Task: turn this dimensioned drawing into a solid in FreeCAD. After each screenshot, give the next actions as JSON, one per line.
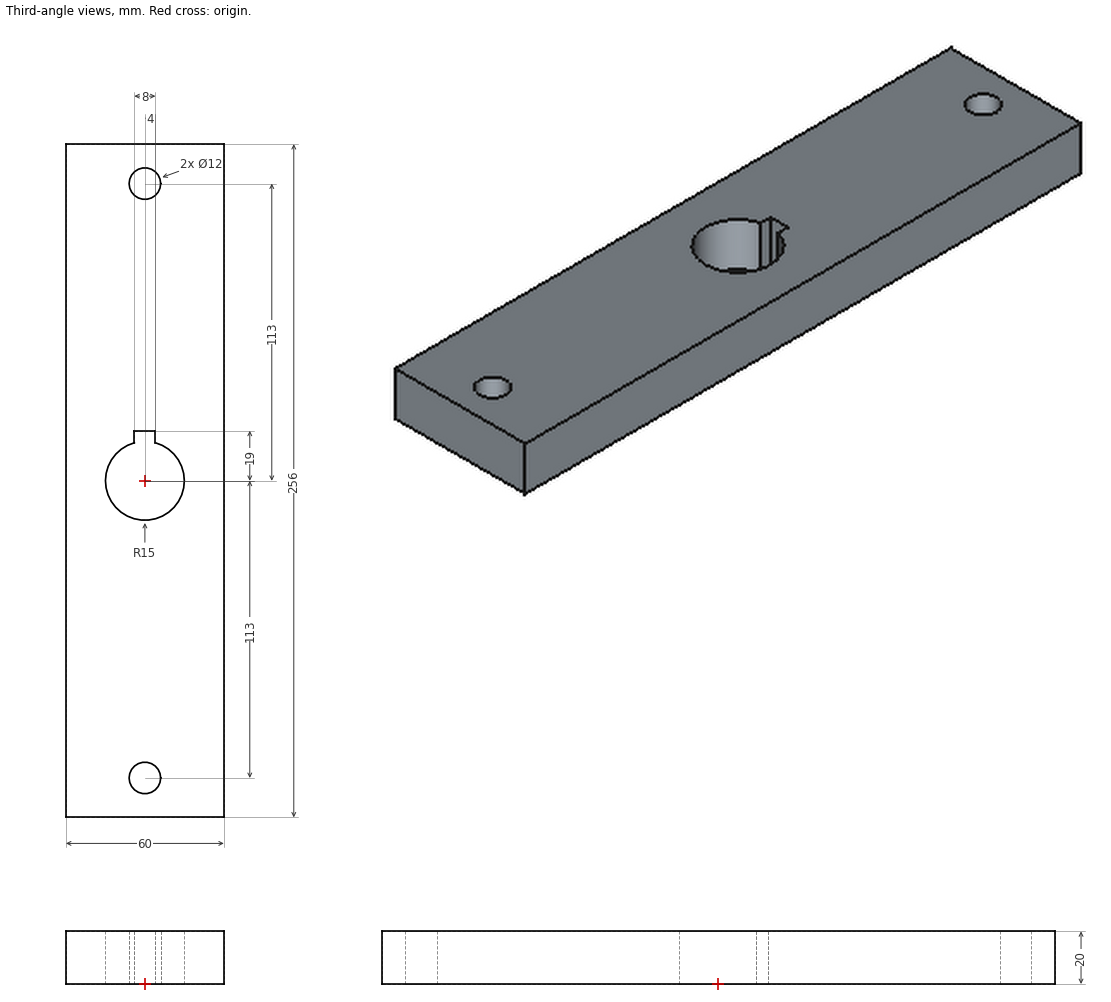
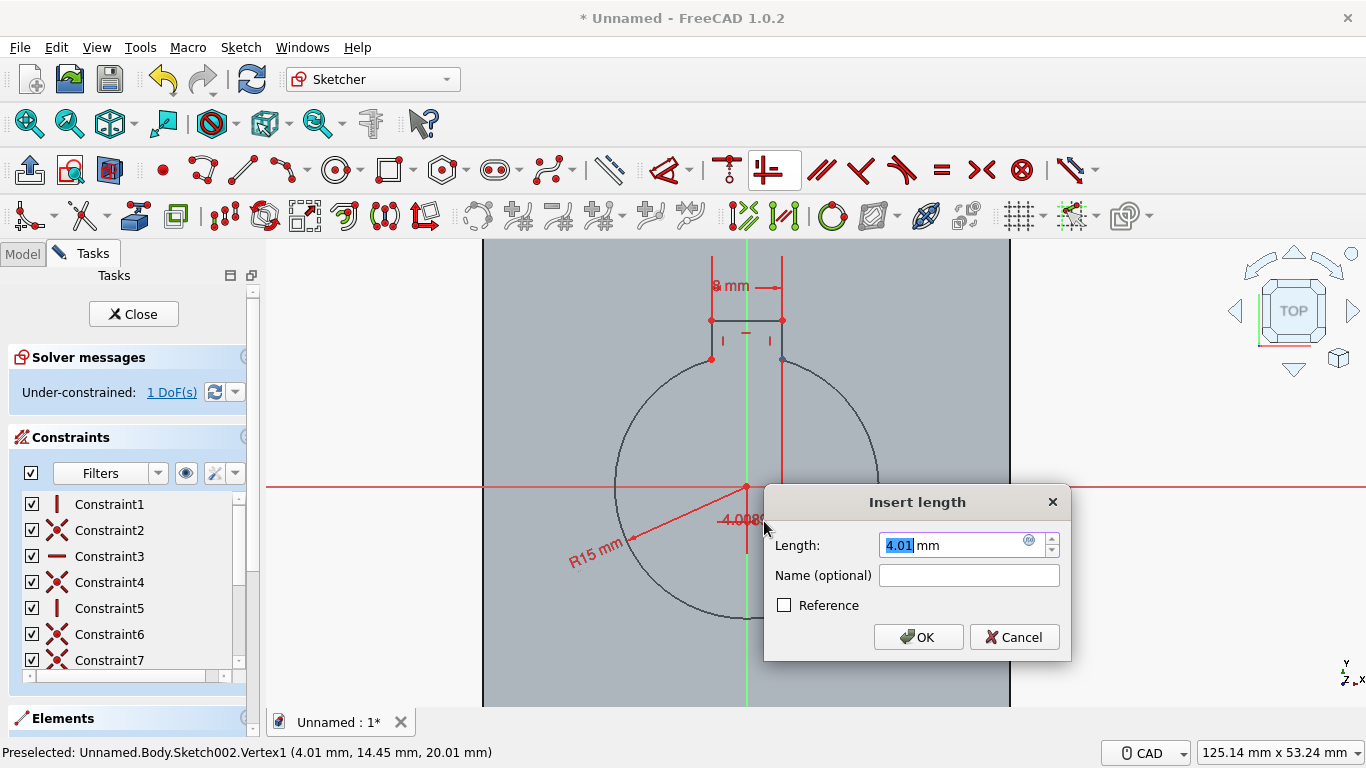
{"action": "type", "text": "4"}
{"action": "key", "text": "Return"}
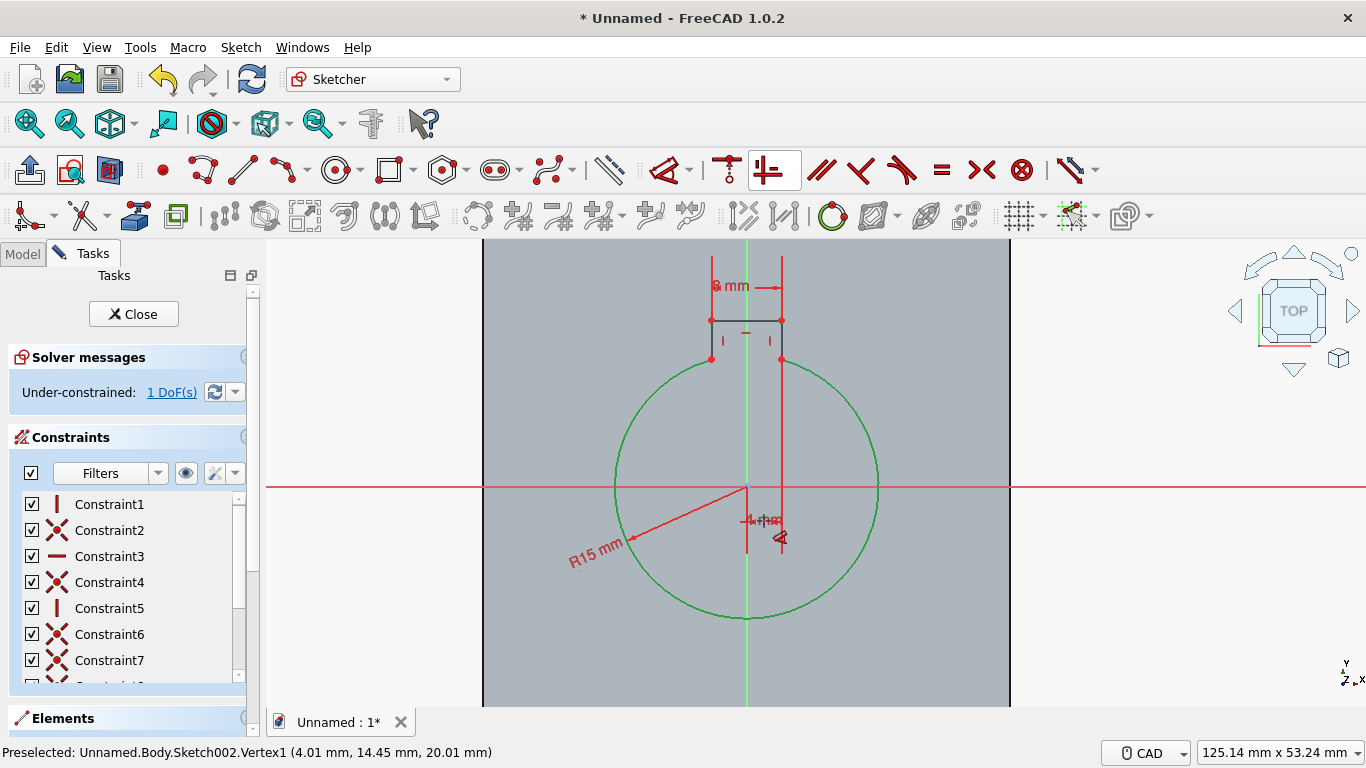
{"action": "left_click", "coordinate": [782, 321]}
{"action": "left_click", "coordinate": [816, 404]}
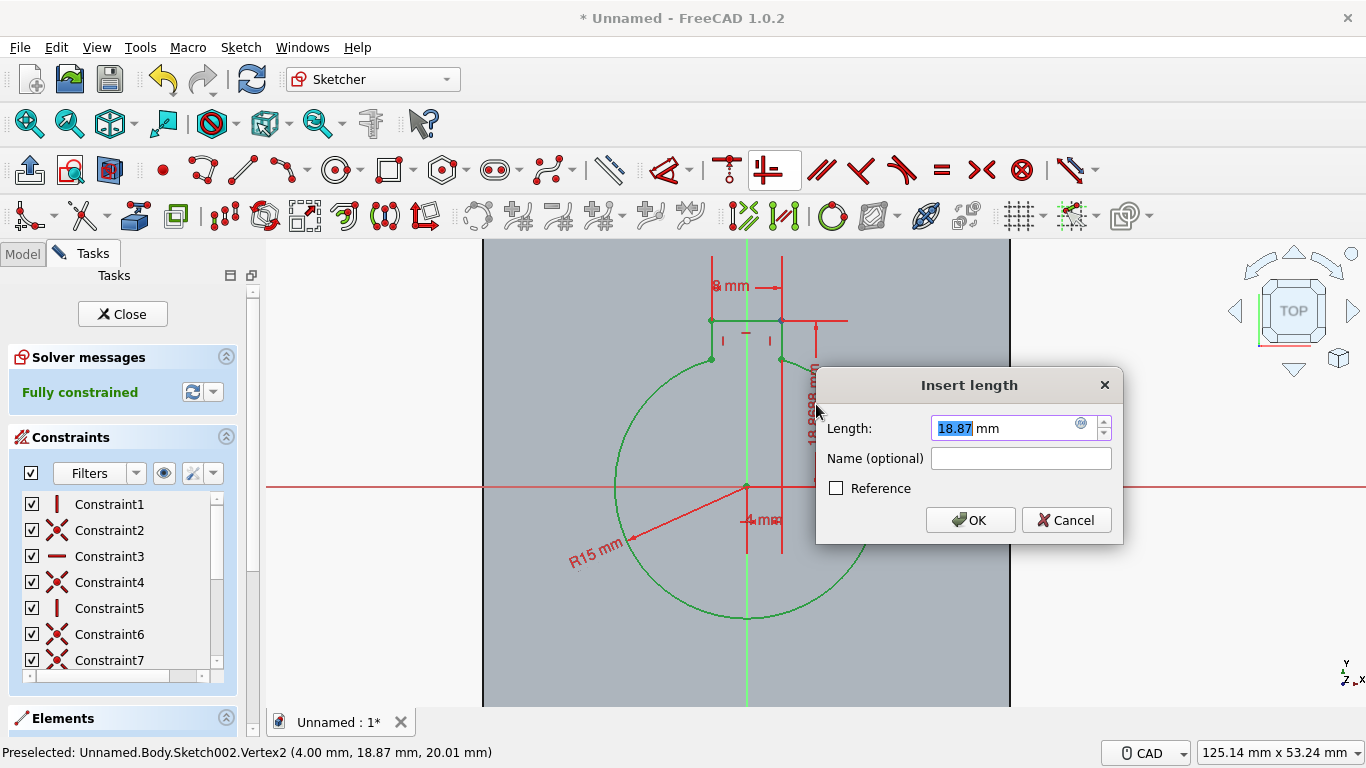
{"action": "type", "text": "19"}
{"action": "key", "text": "Return"}
{"action": "key", "text": "Escape"}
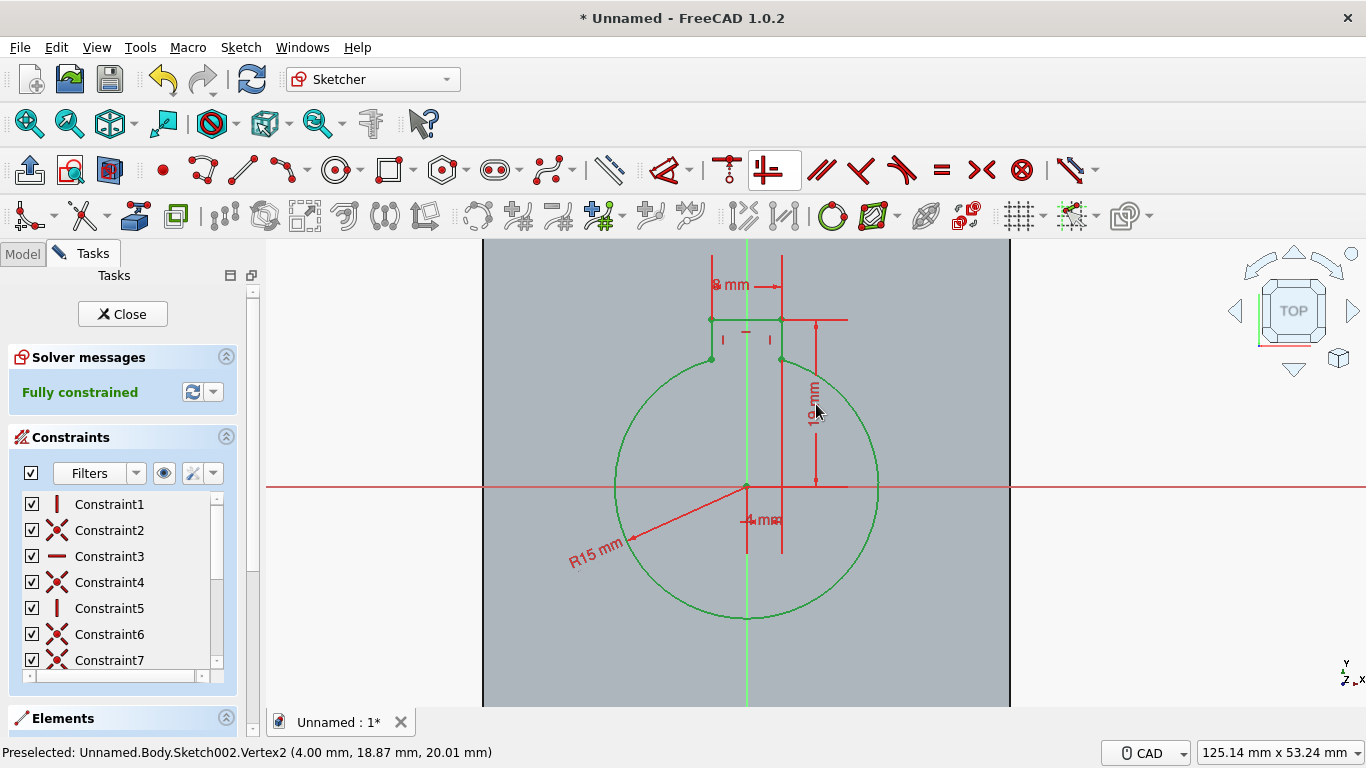
{"action": "left_click", "coordinate": [123, 314]}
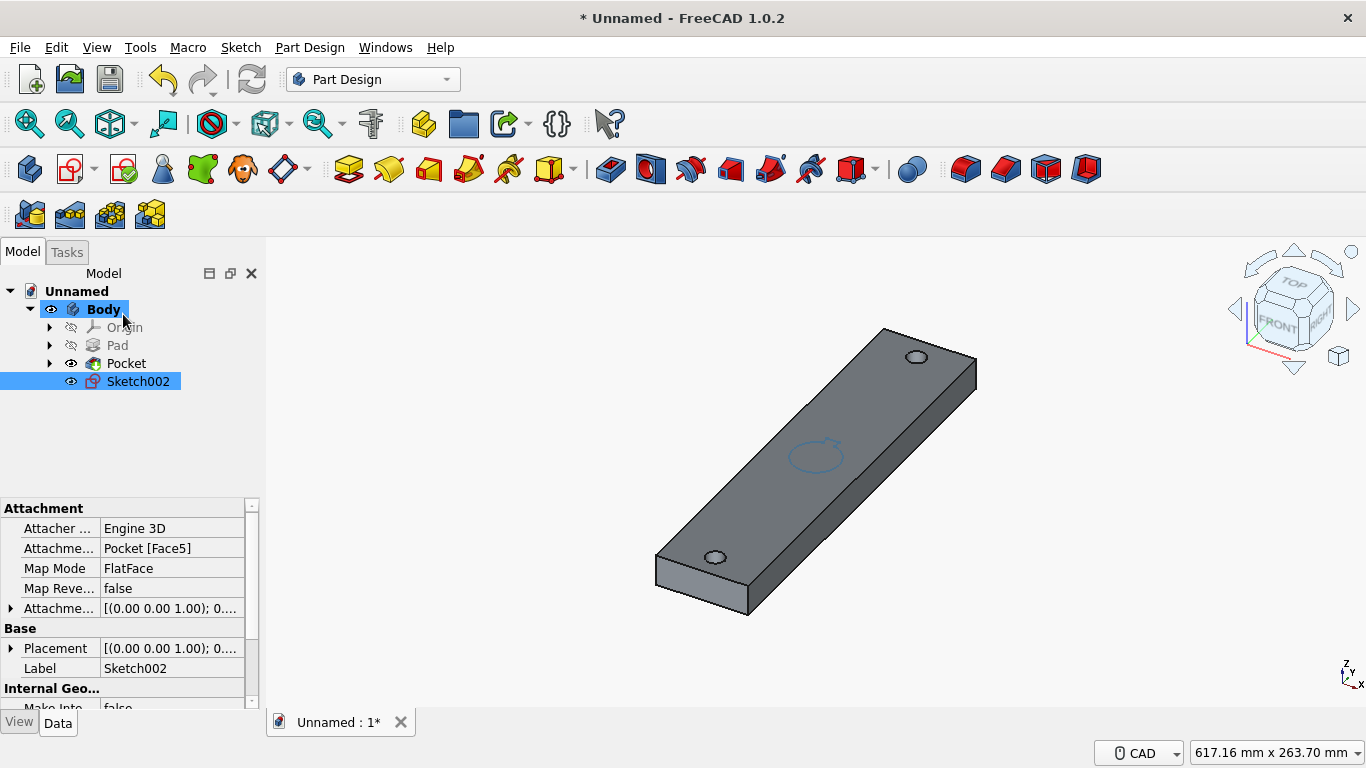
{"action": "left_click", "coordinate": [612, 170]}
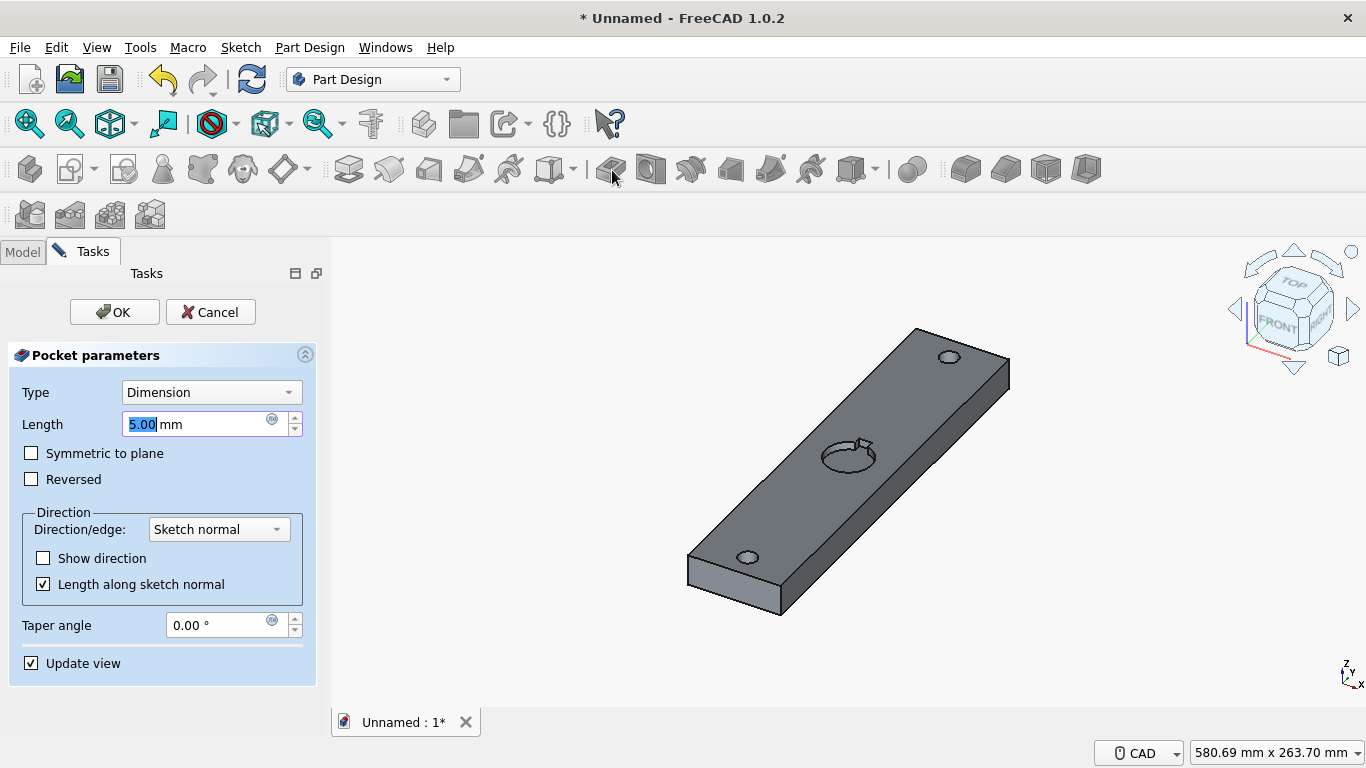
{"action": "left_click", "coordinate": [212, 392]}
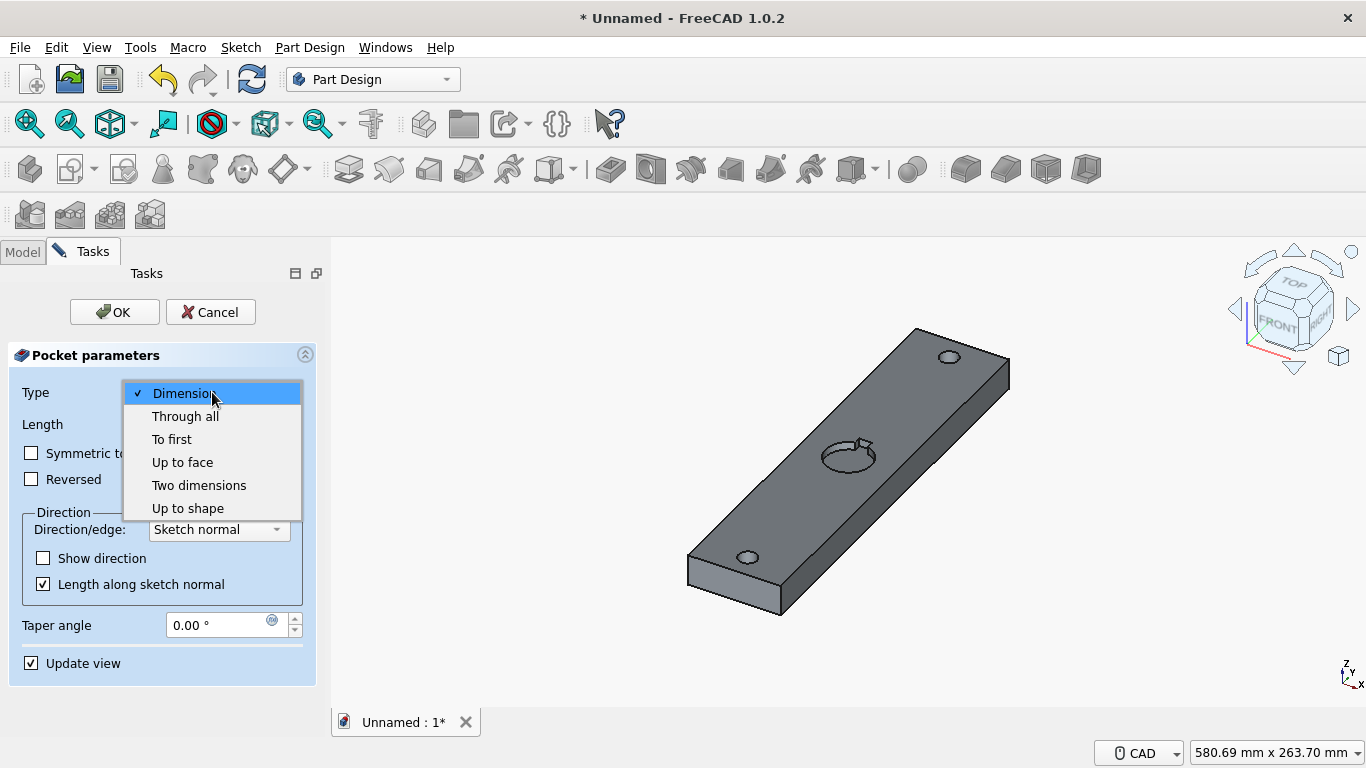
{"action": "left_click", "coordinate": [212, 416]}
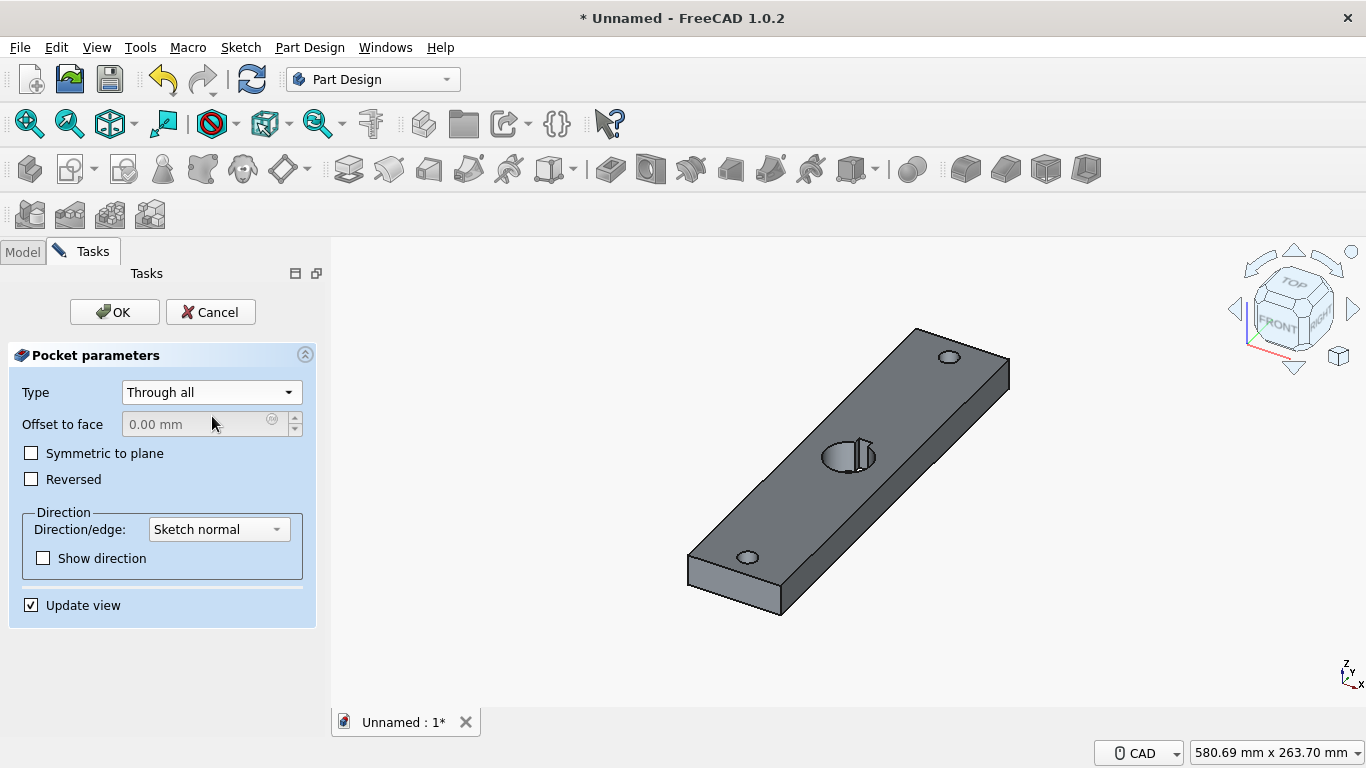
{"action": "left_click", "coordinate": [115, 312]}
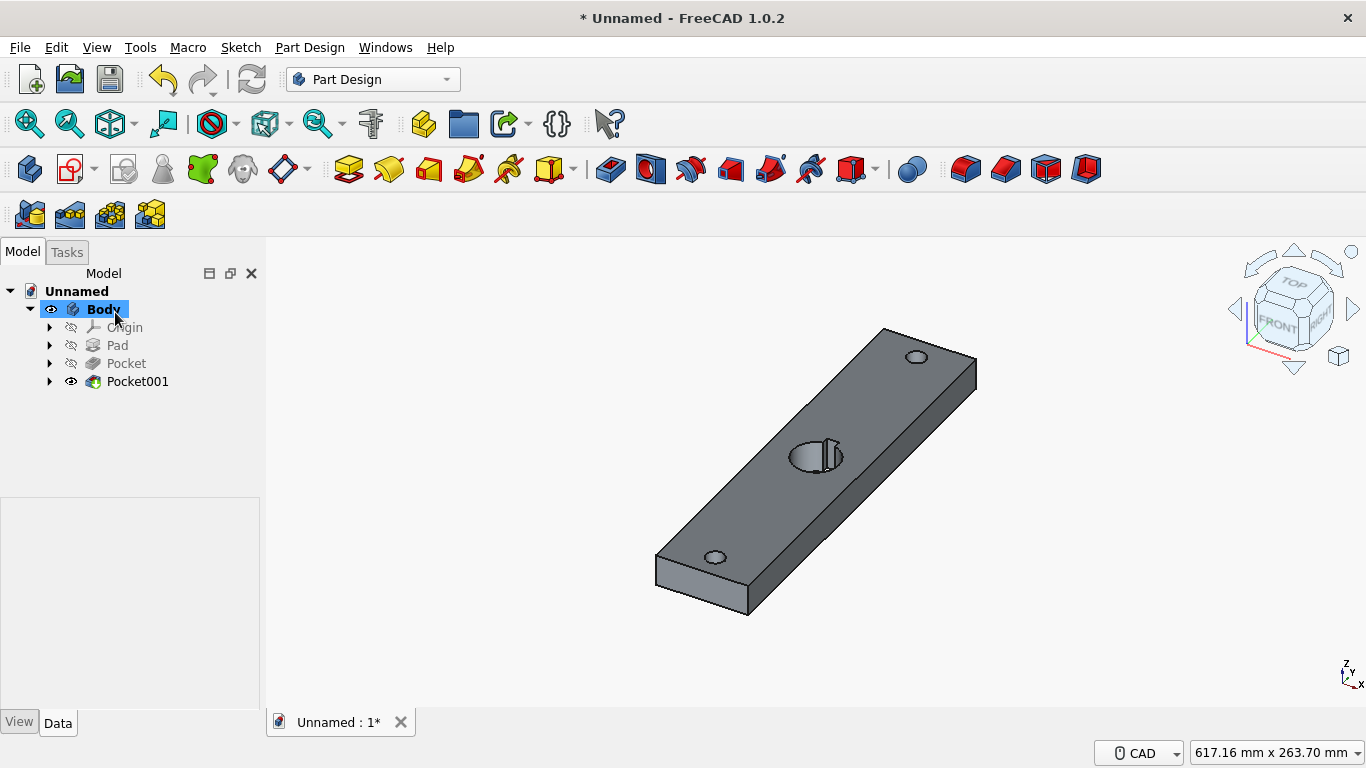
{"action": "key", "text": "0"}